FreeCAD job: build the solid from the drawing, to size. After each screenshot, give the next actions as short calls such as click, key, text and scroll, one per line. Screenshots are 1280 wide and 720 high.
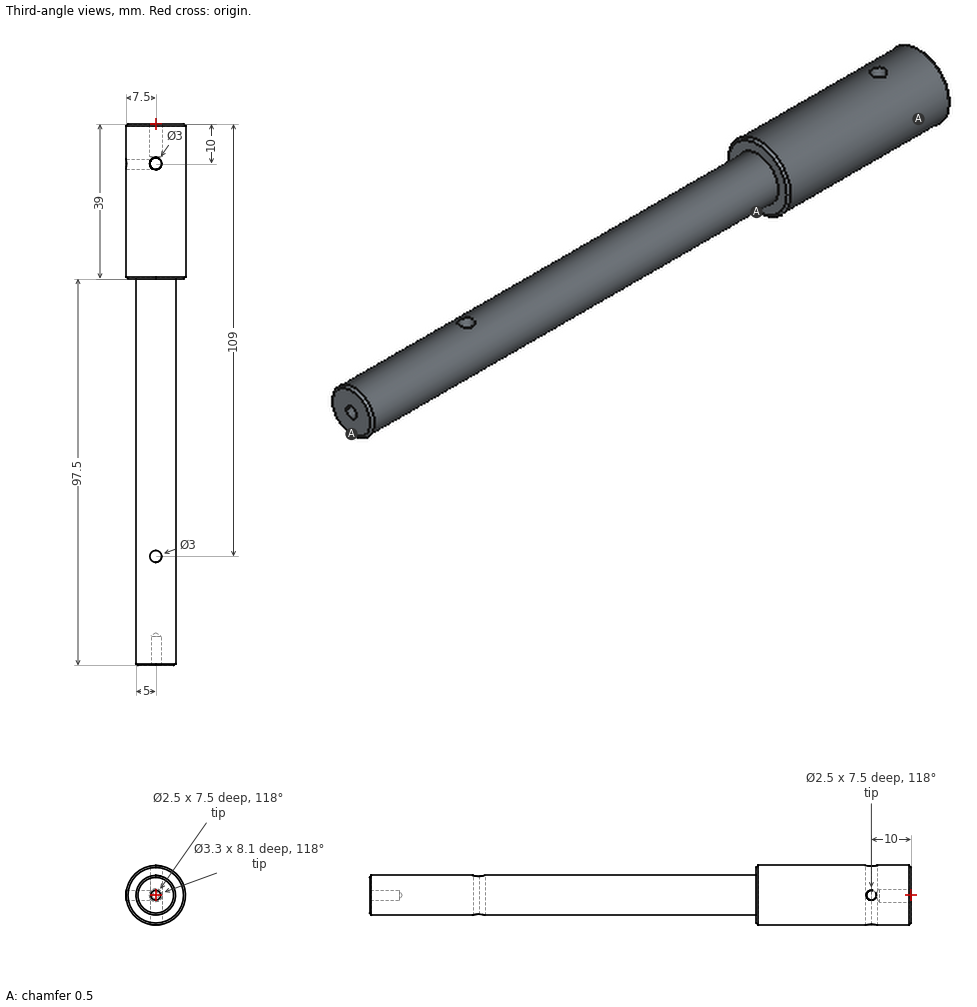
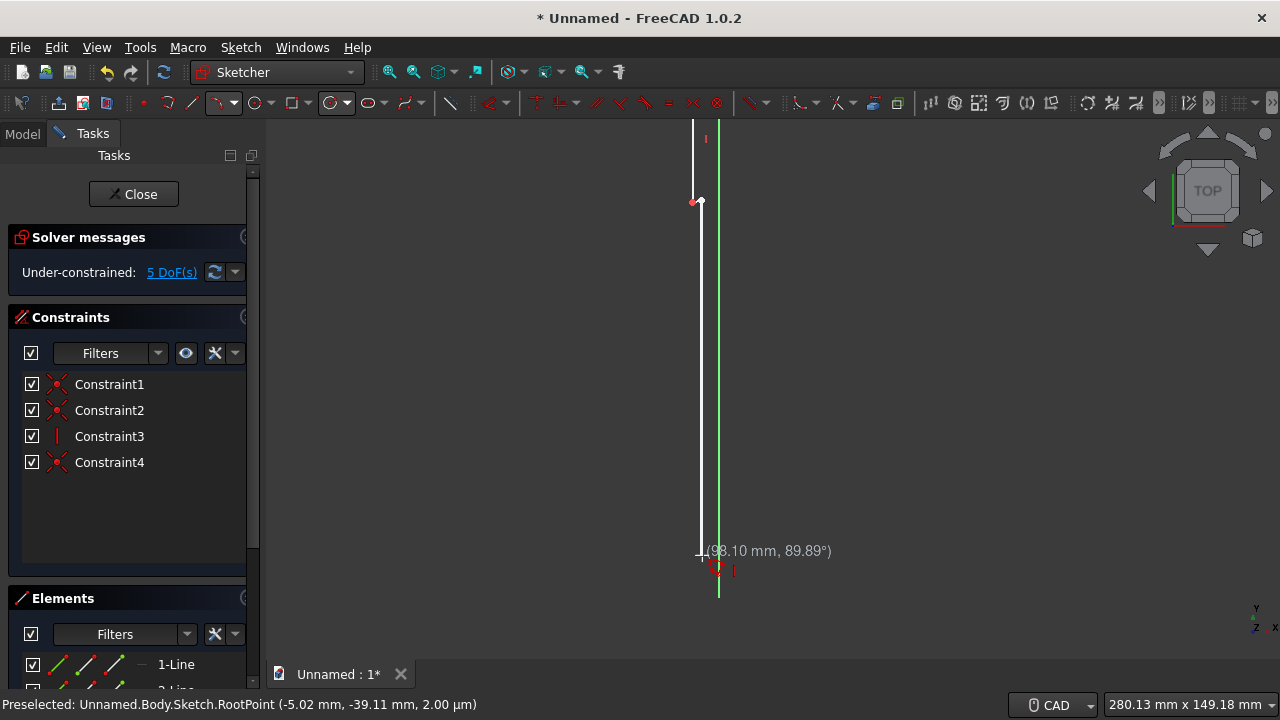
click(701, 554)
click(710, 554)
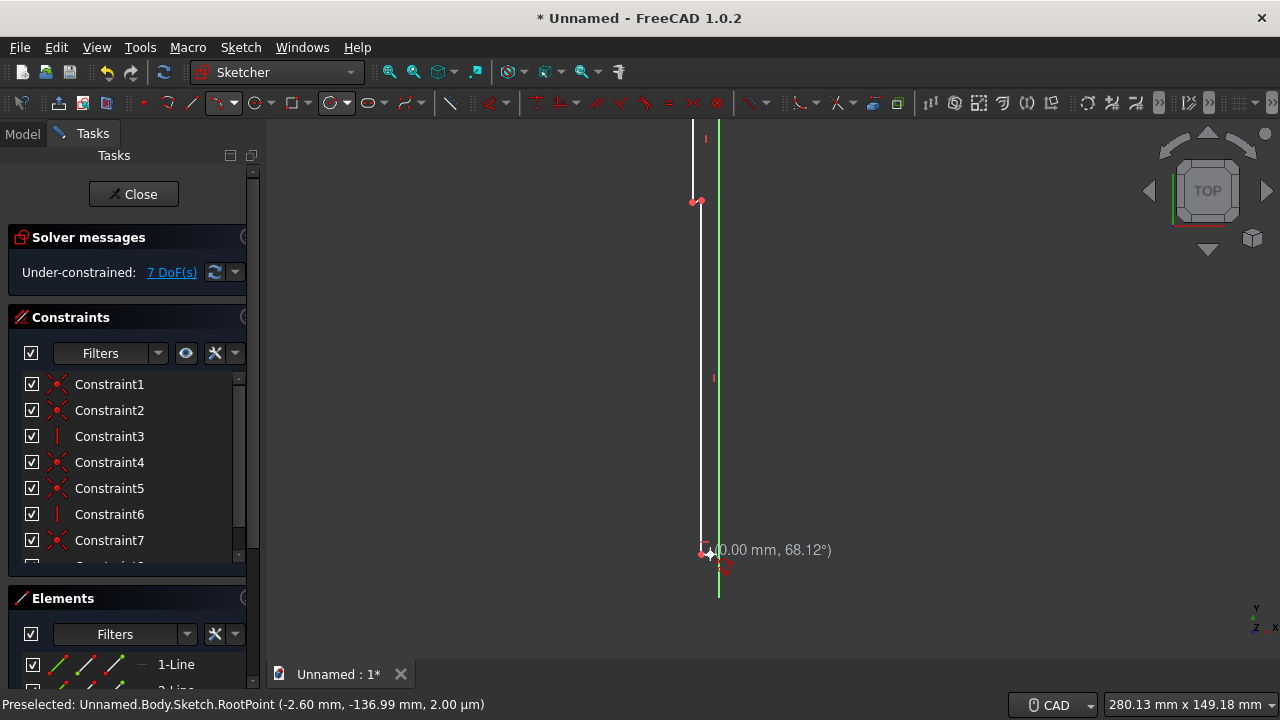
scroll(702, 556, down, 2)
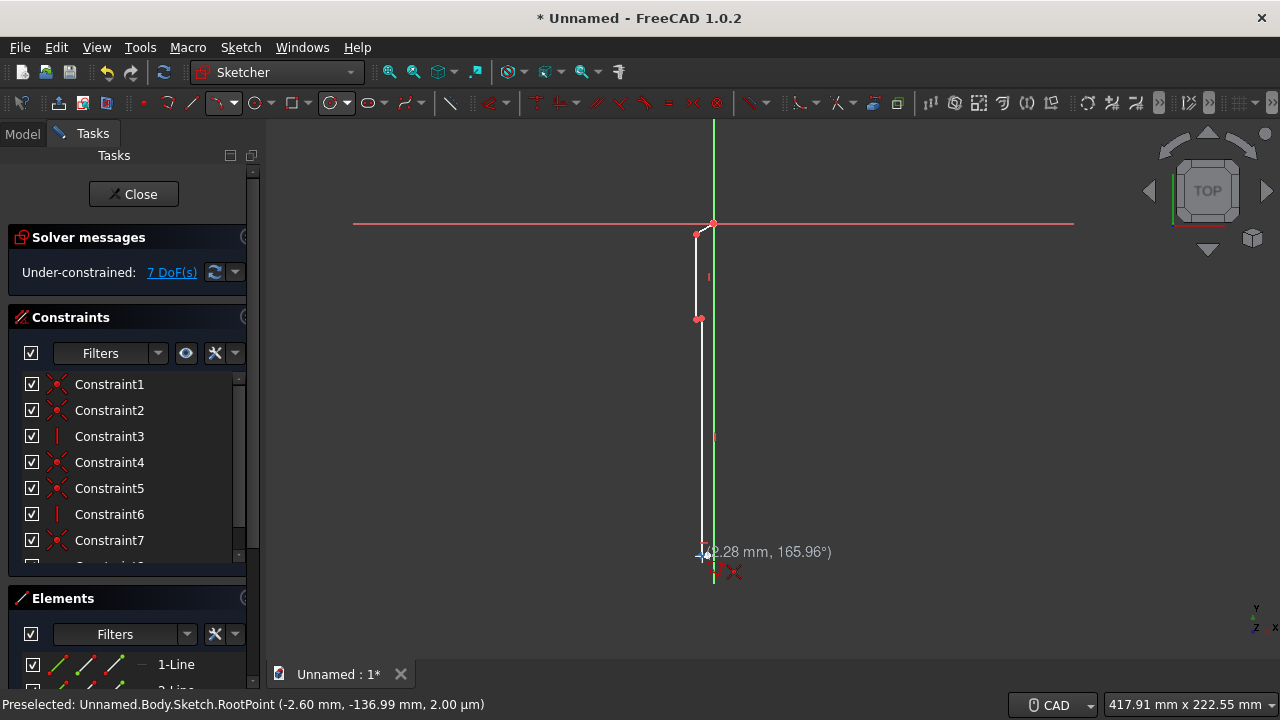
scroll(714, 224, up, 3)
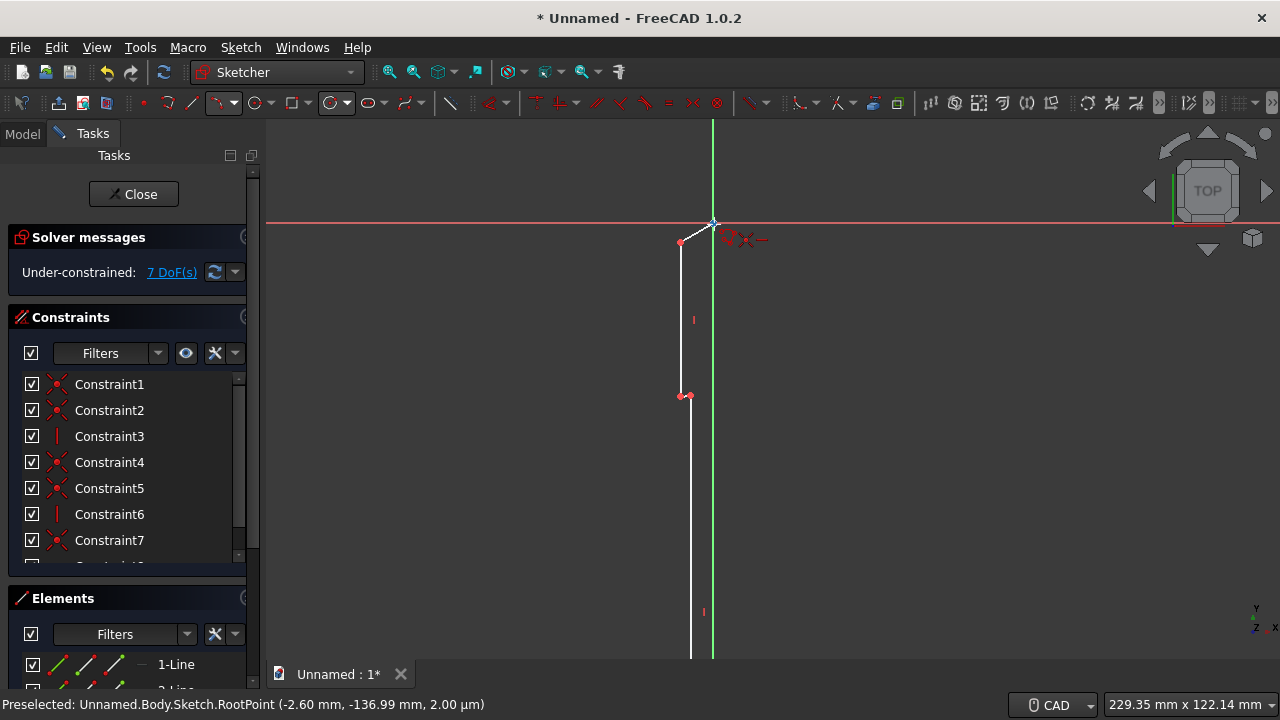
click(713, 223)
key(Escape)
key(Escape)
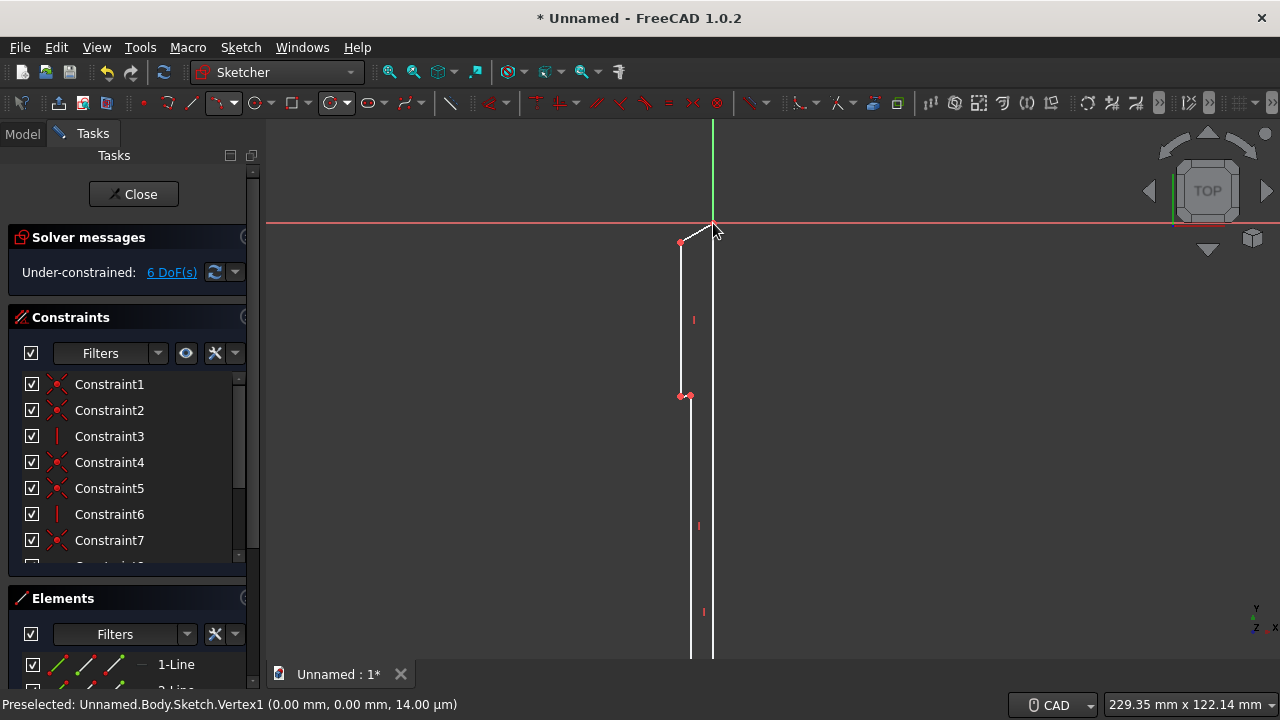
scroll(691, 237, up, 2)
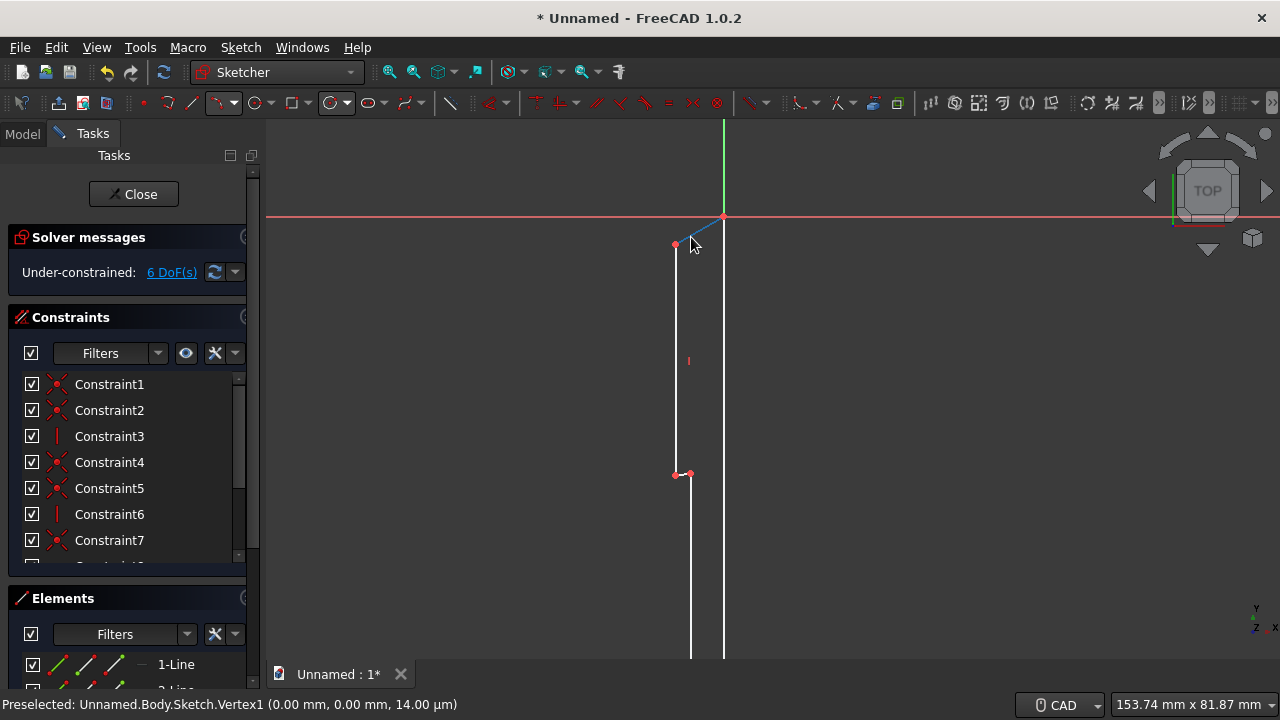
click(690, 236)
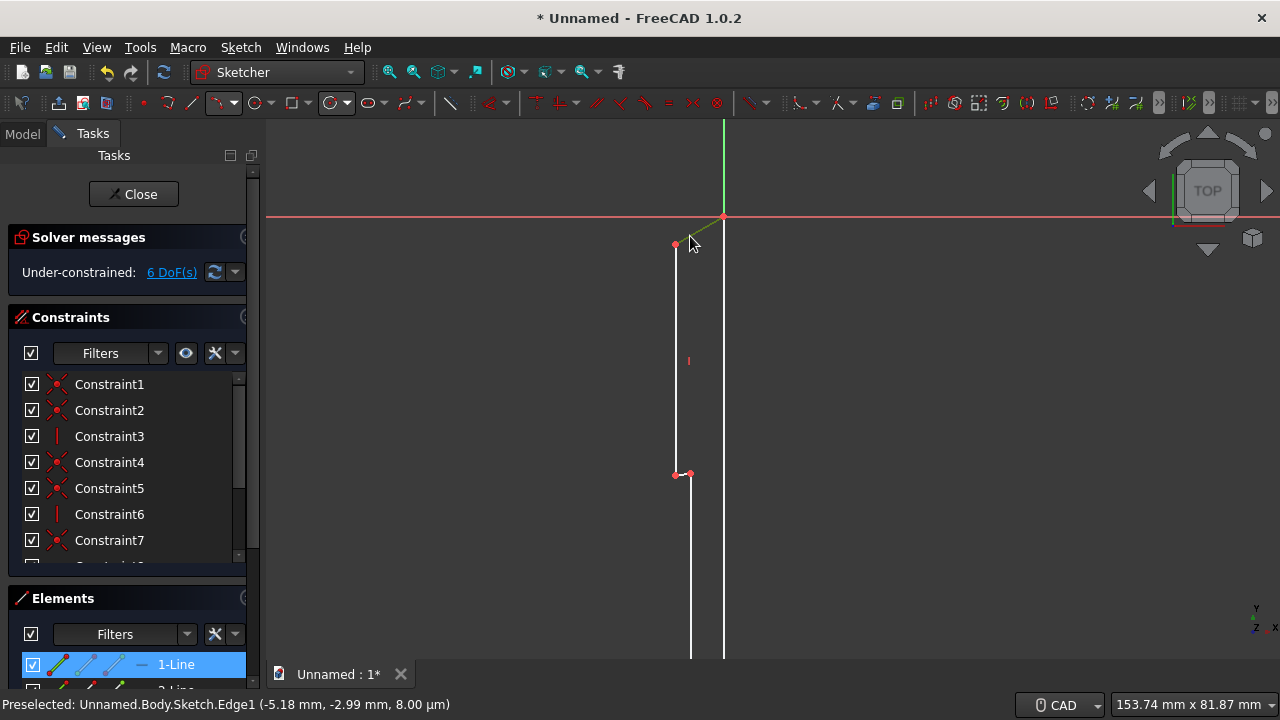
click(578, 104)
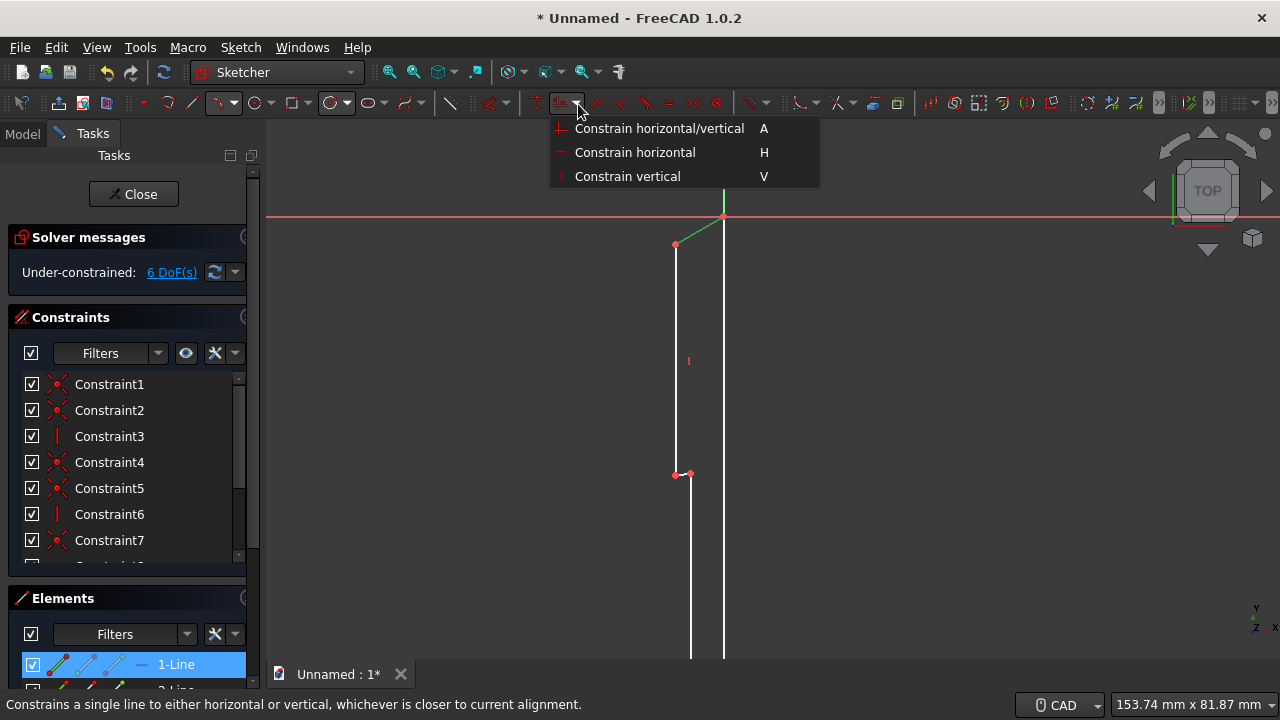
click(685, 152)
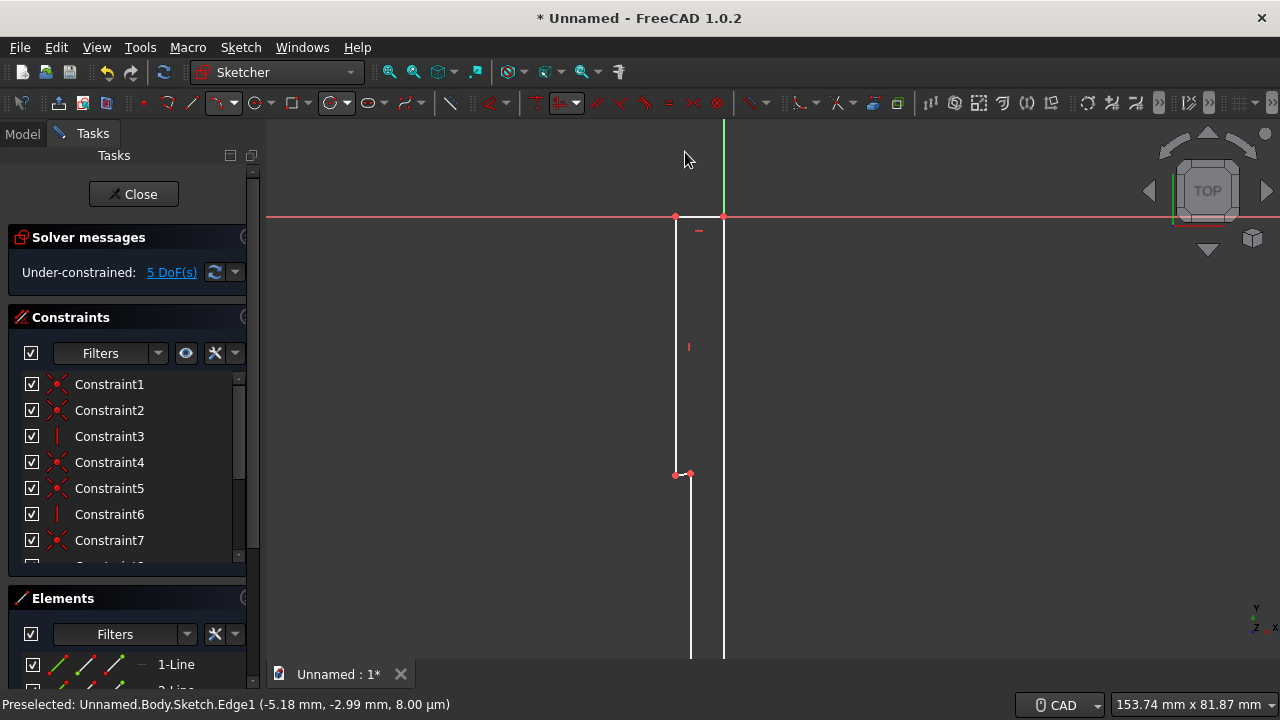
scroll(683, 475, up, 4)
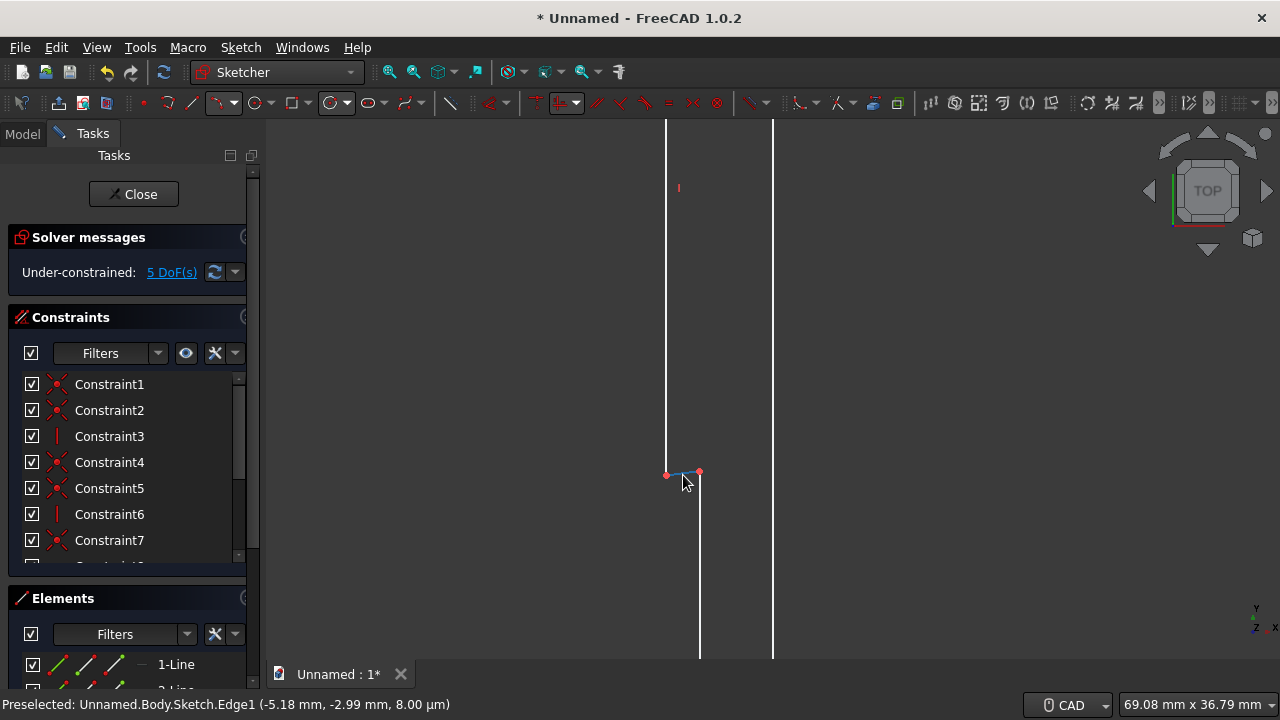
click(683, 473)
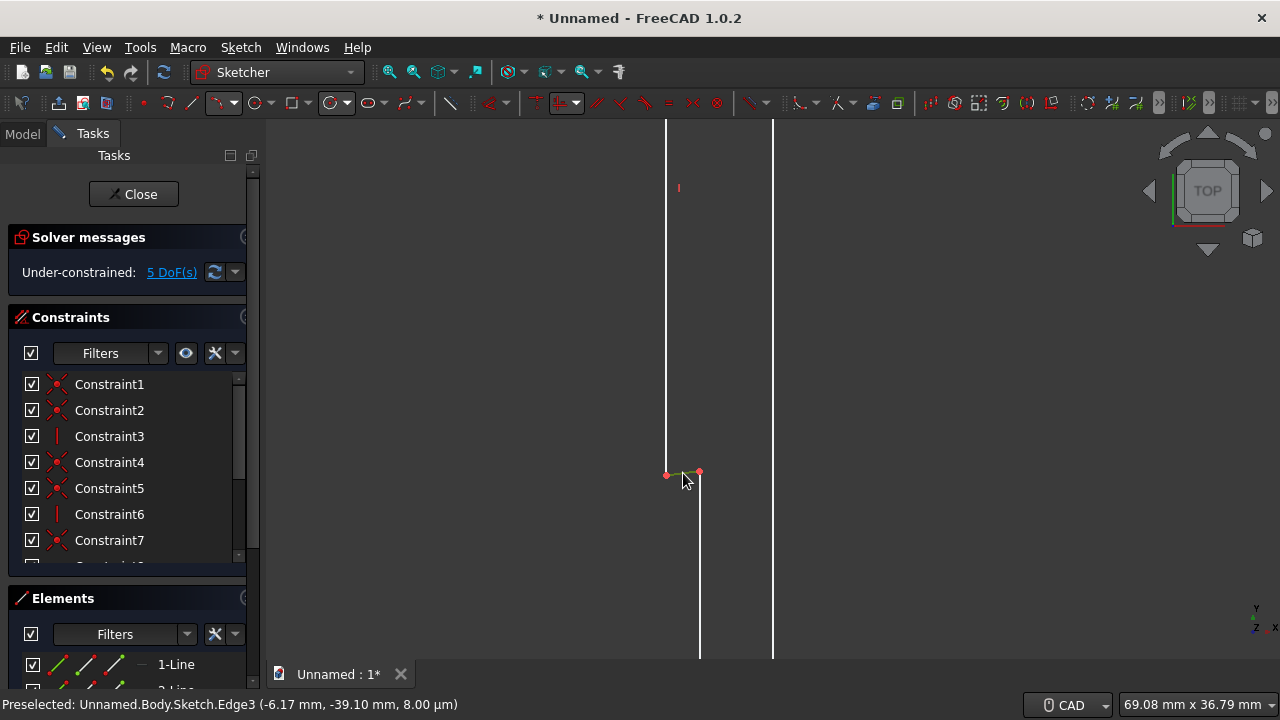
key(h)